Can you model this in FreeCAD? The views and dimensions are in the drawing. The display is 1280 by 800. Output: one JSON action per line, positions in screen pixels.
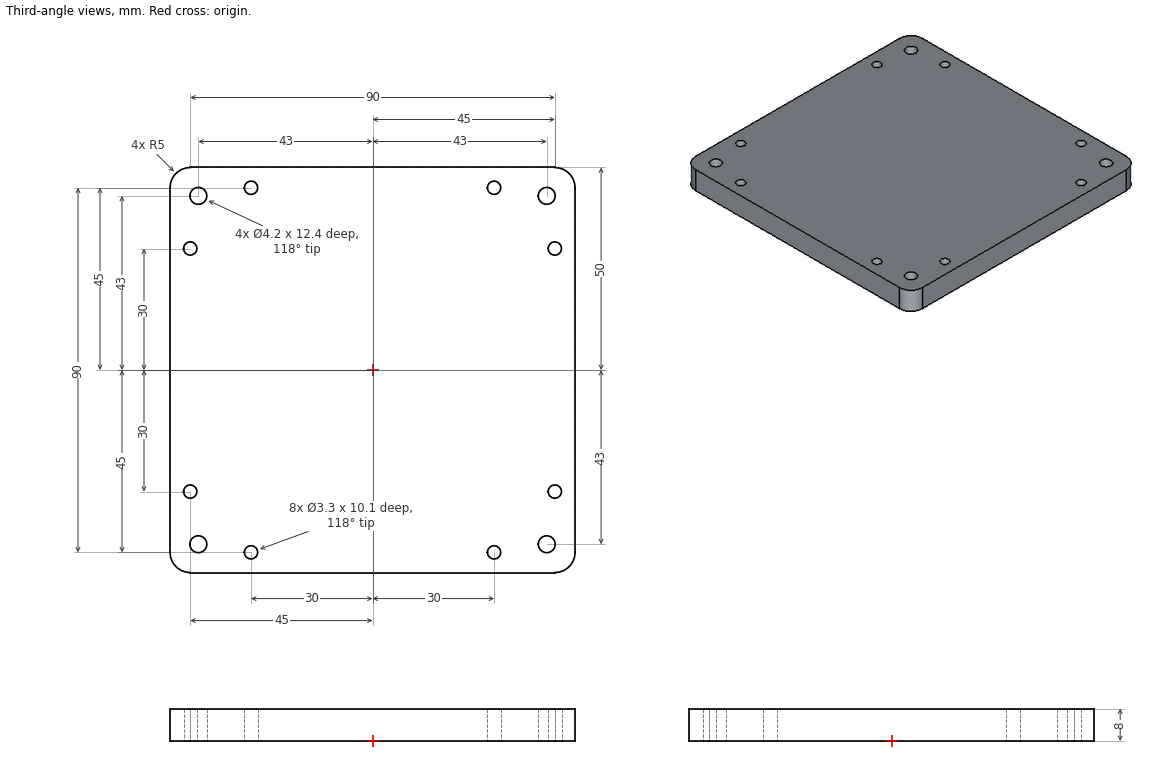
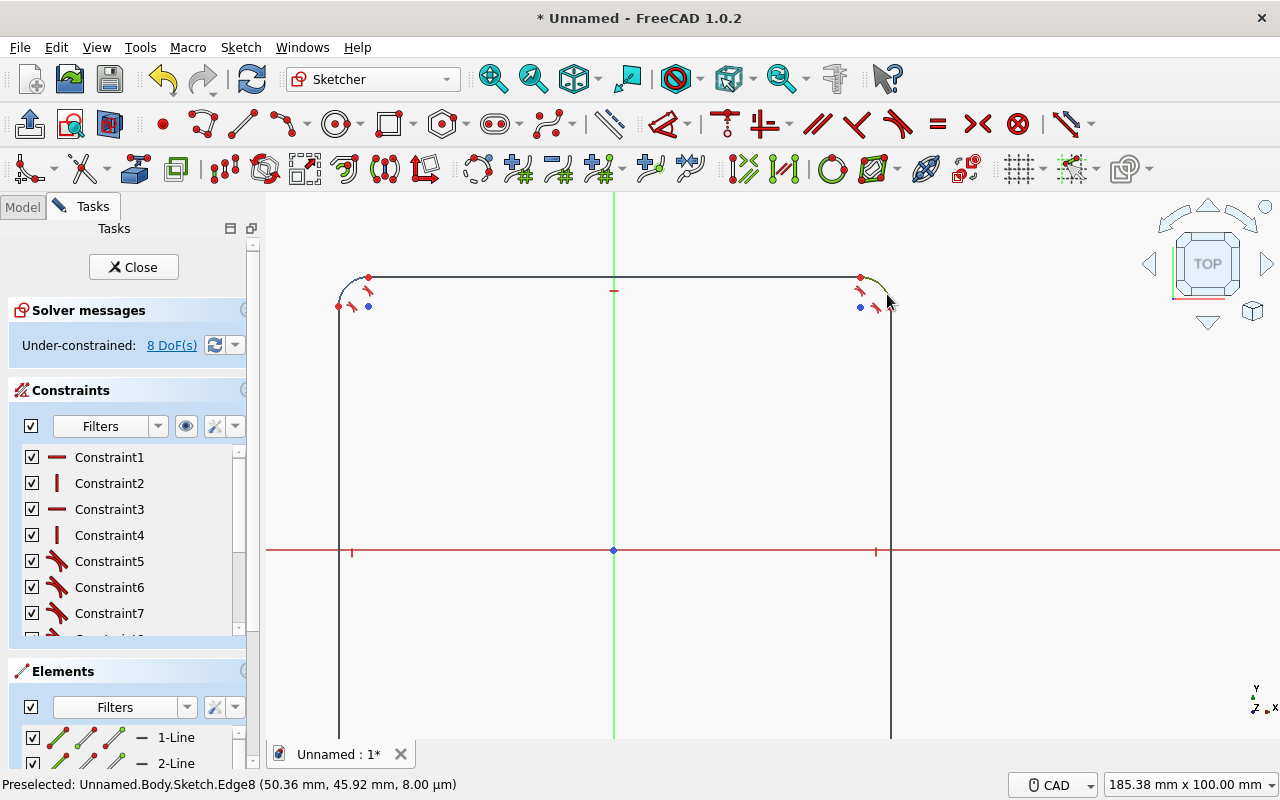
{"action": "key", "text": "e"}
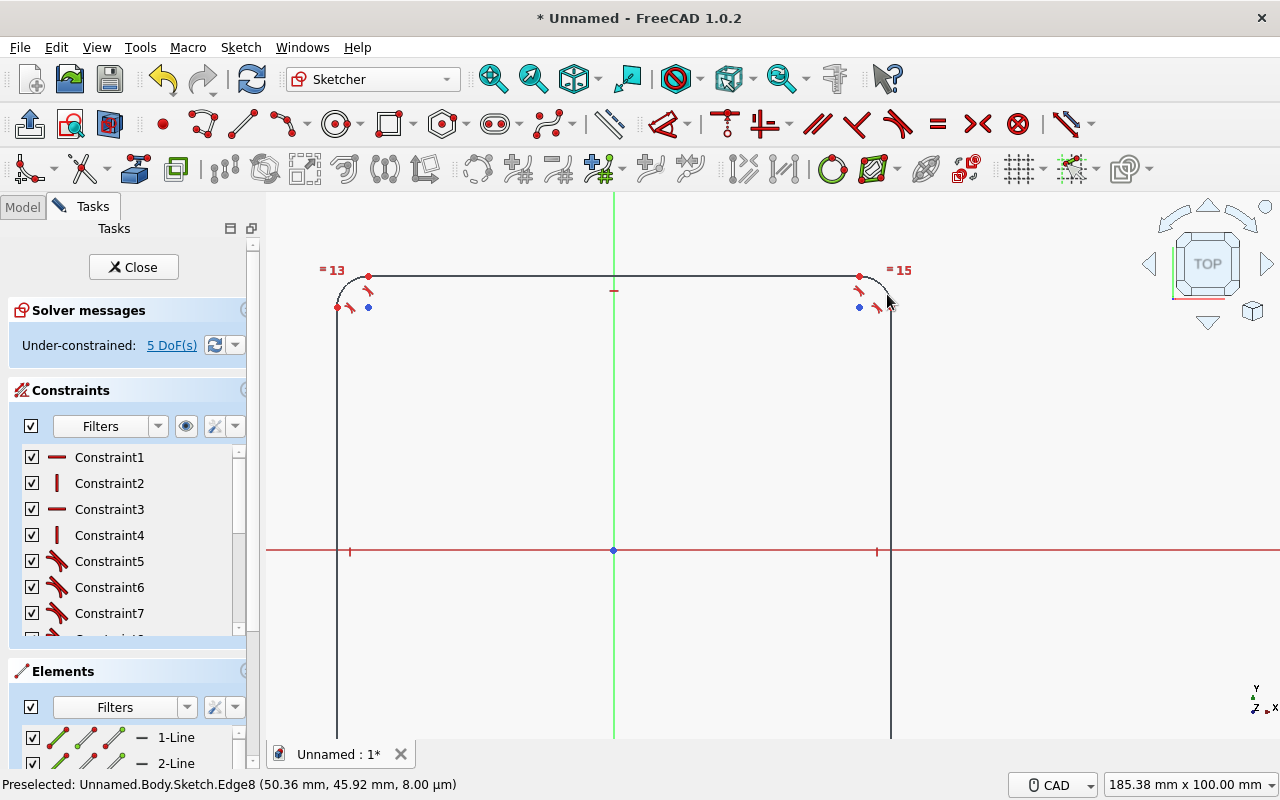
{"action": "key", "text": "d"}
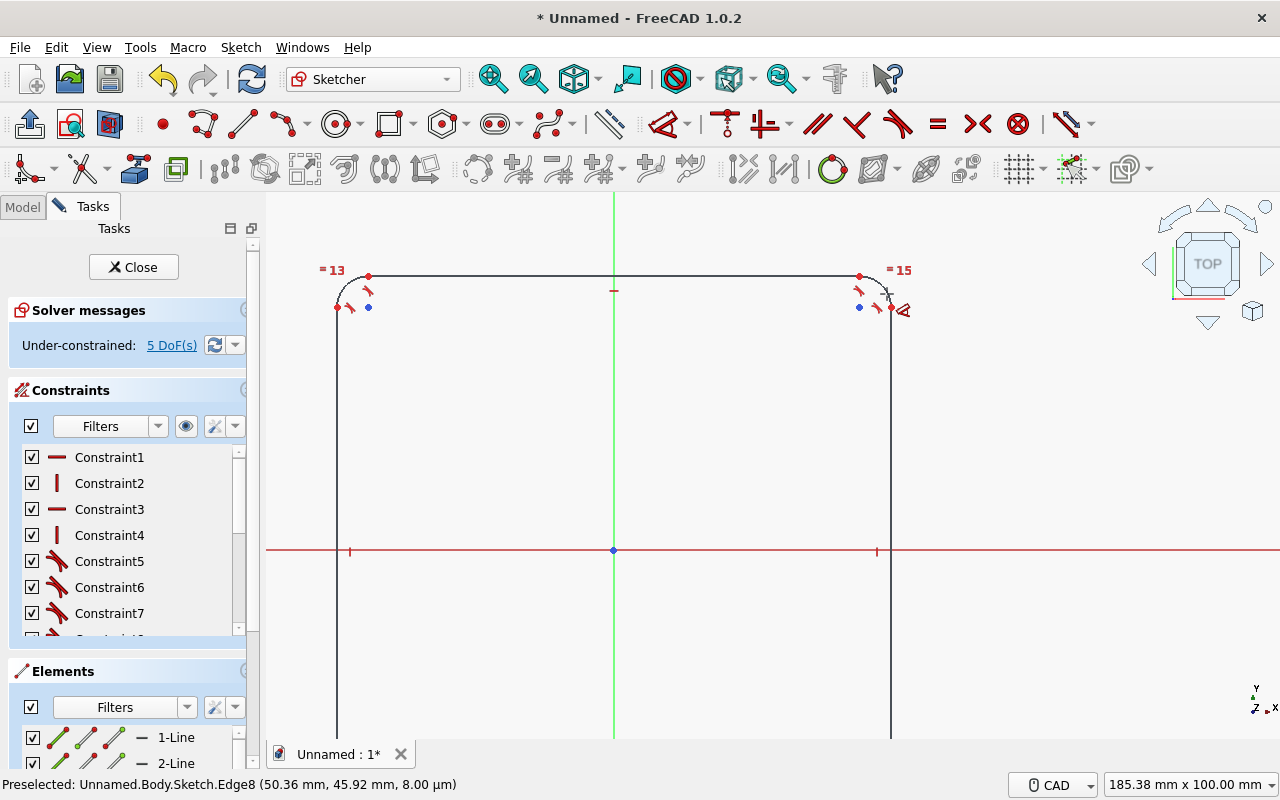
{"action": "scroll", "coordinate": [354, 280], "scroll_direction": "up", "scroll_amount": 2}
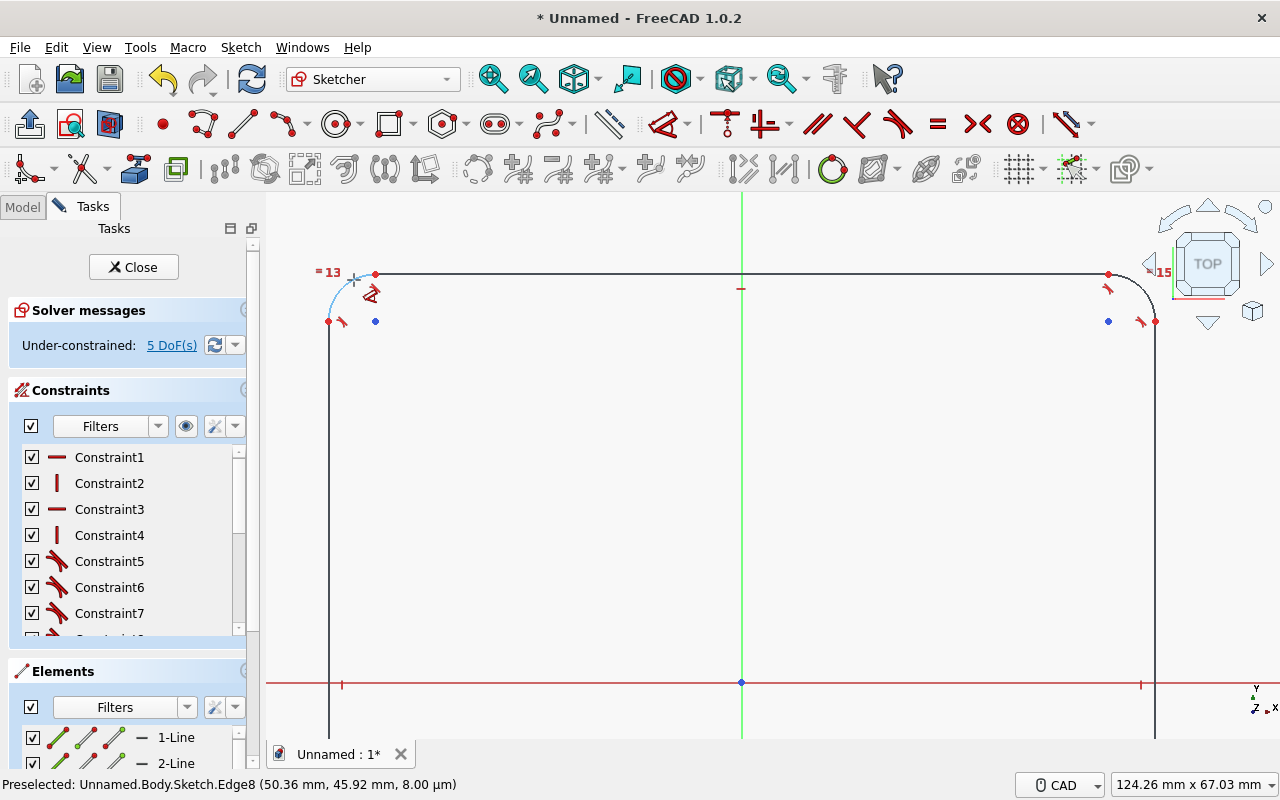
{"action": "left_click", "coordinate": [354, 280]}
{"action": "left_click", "coordinate": [339, 252]}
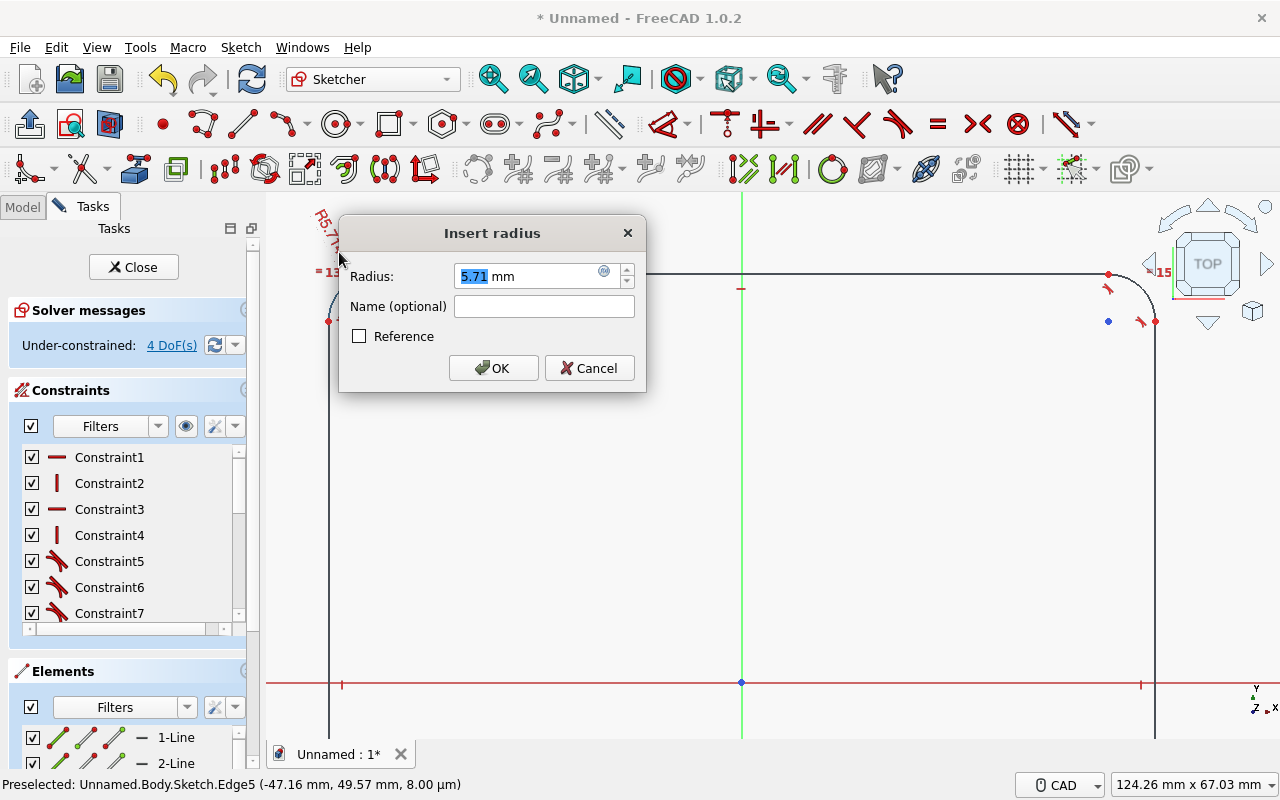
{"action": "type", "text": "5"}
{"action": "key", "text": "Return"}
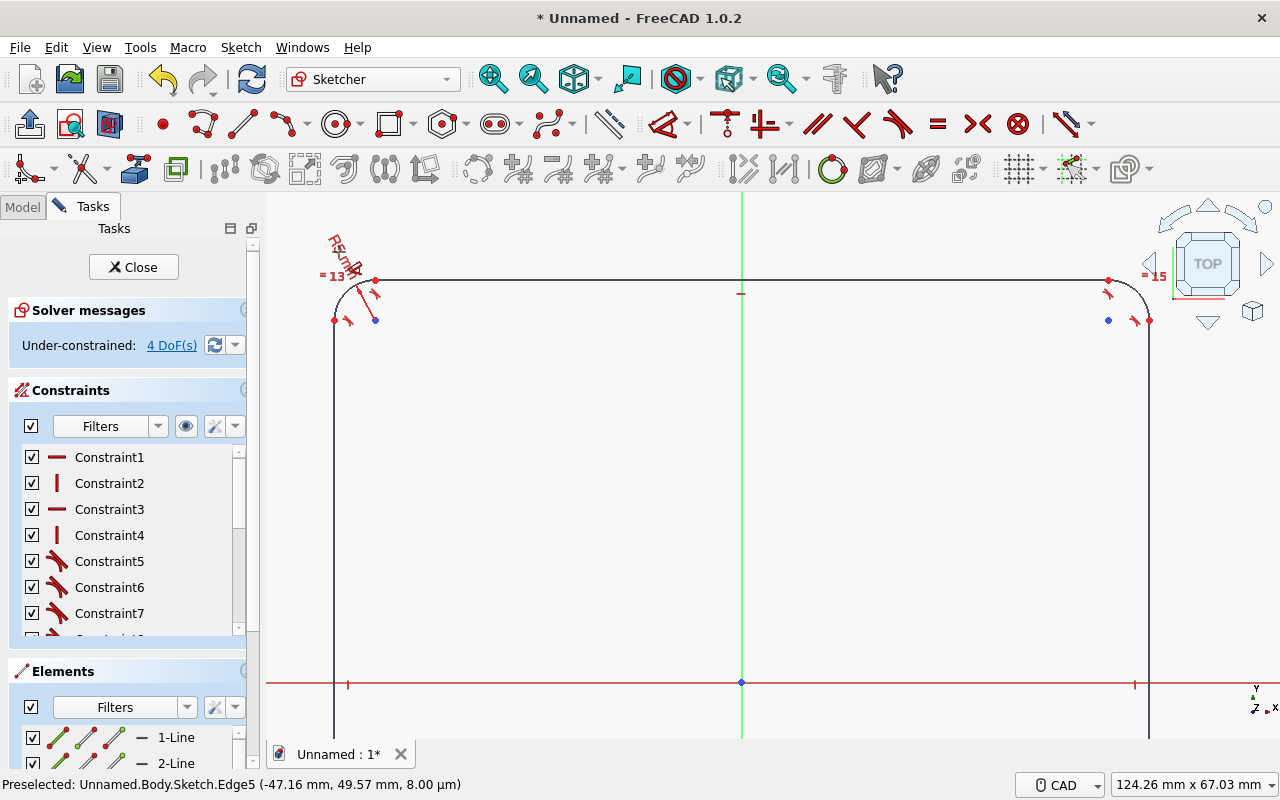
{"action": "left_click", "coordinate": [889, 280]}
{"action": "left_click", "coordinate": [573, 246]}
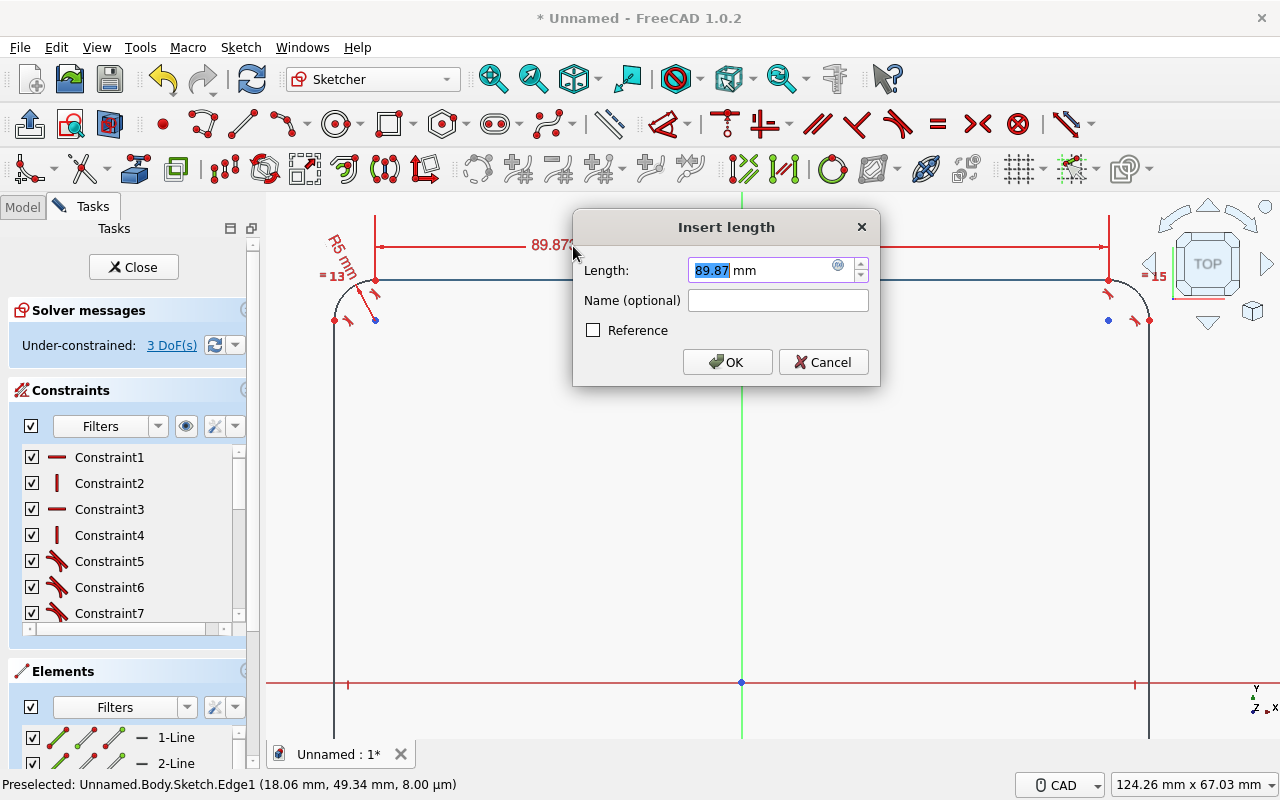
{"action": "type", "text": "90"}
{"action": "key", "text": "Return"}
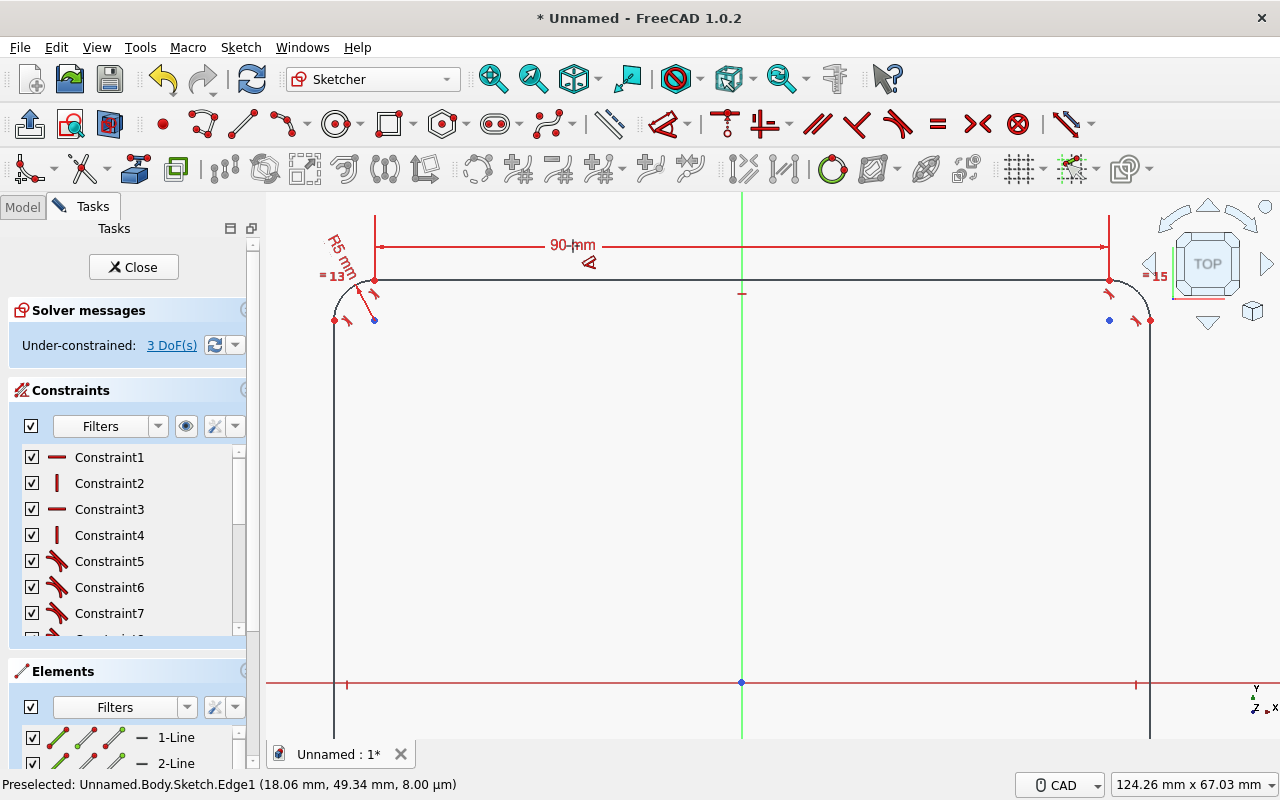
{"action": "left_click", "coordinate": [334, 539]}
{"action": "left_click", "coordinate": [300, 516]}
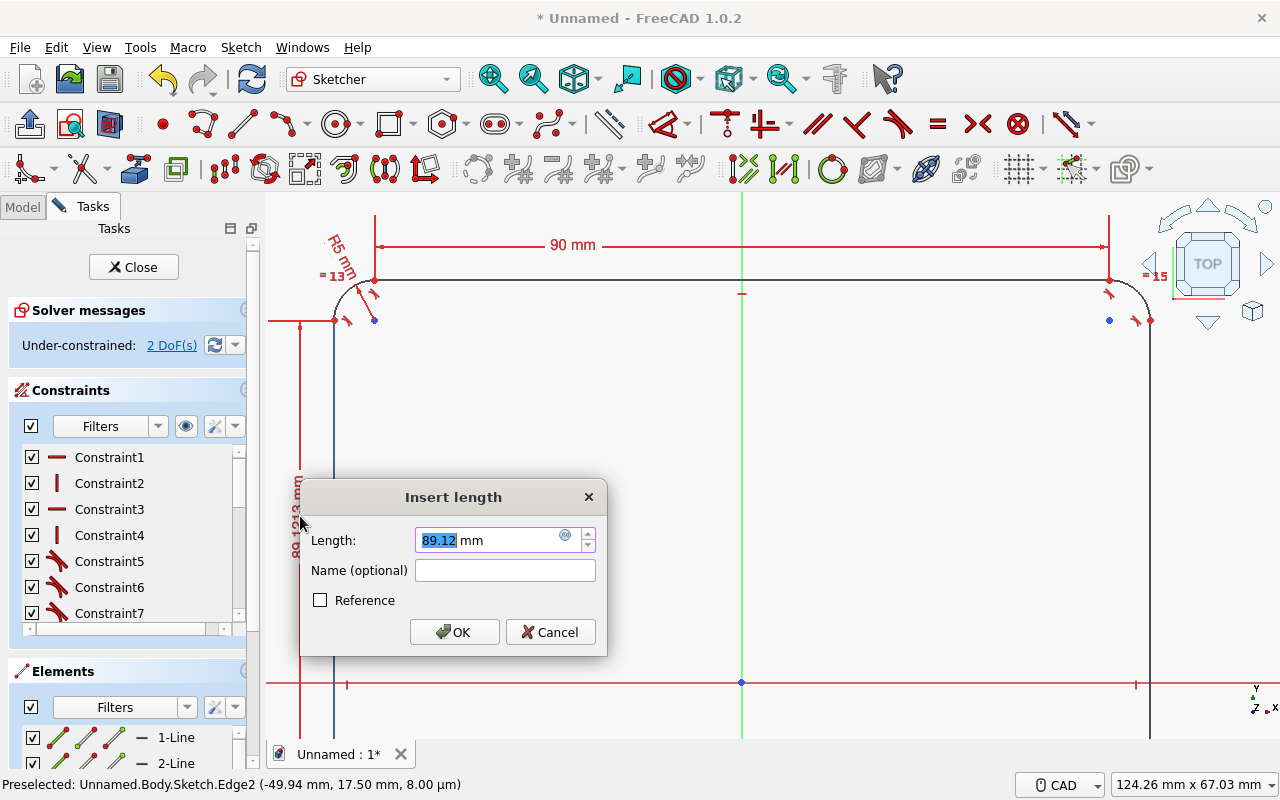
{"action": "type", "text": "90"}
{"action": "key", "text": "Return"}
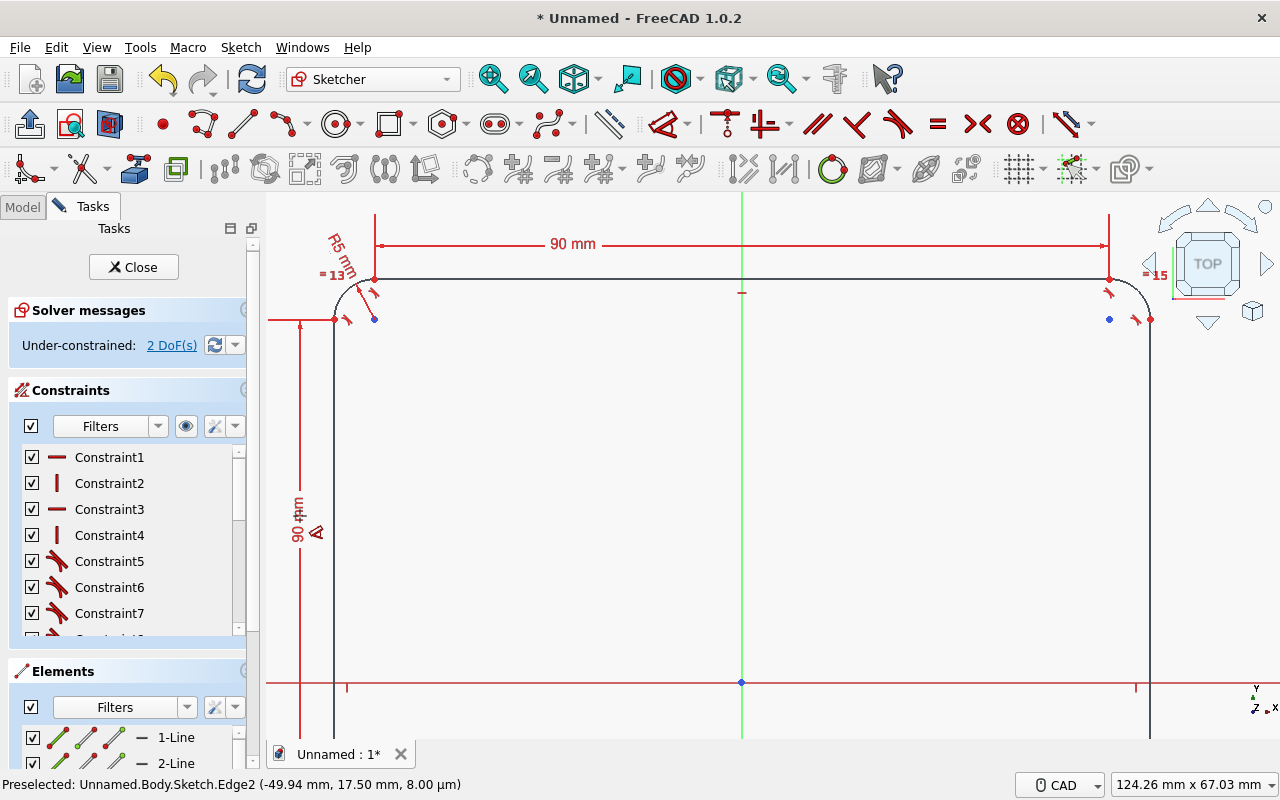
{"action": "left_click", "coordinate": [1109, 279]}
{"action": "left_click", "coordinate": [926, 245]}